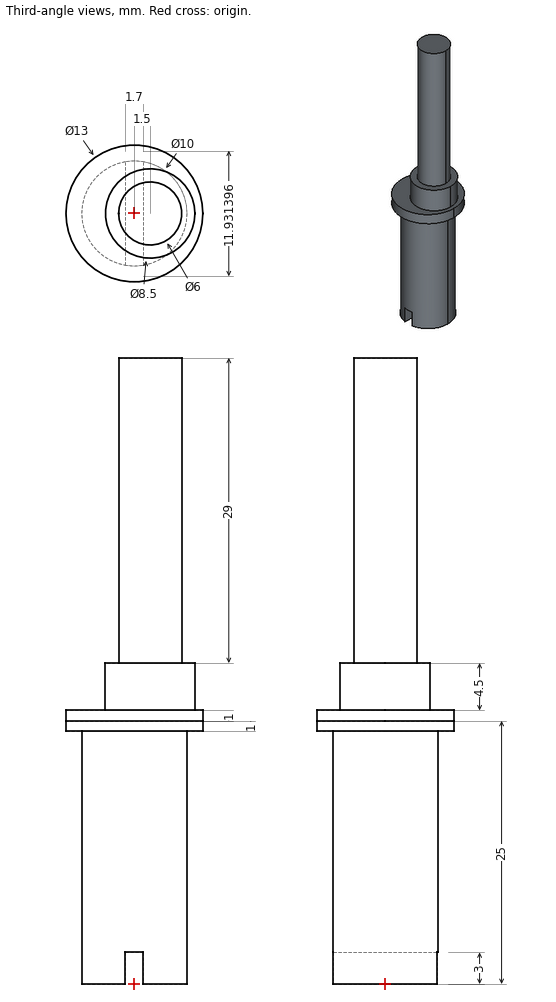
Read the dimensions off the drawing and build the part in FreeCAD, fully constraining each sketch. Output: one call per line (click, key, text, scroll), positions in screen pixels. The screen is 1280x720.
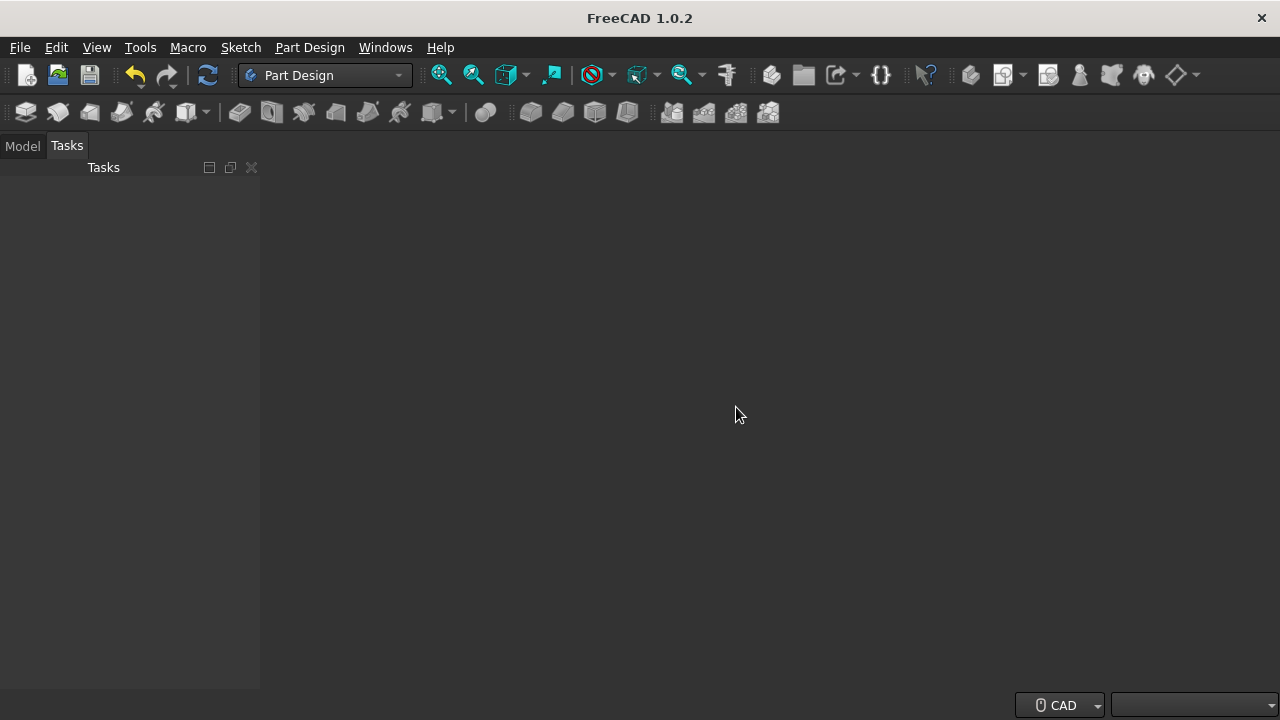
click(26, 76)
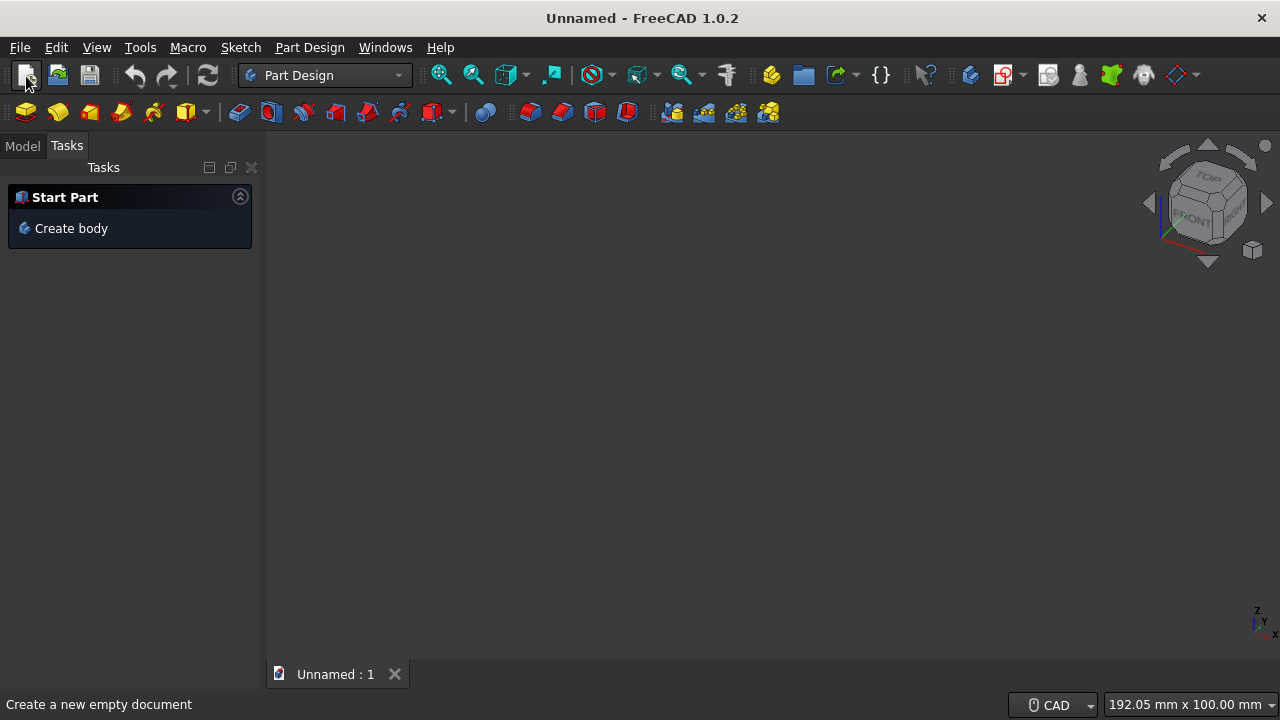
click(1004, 76)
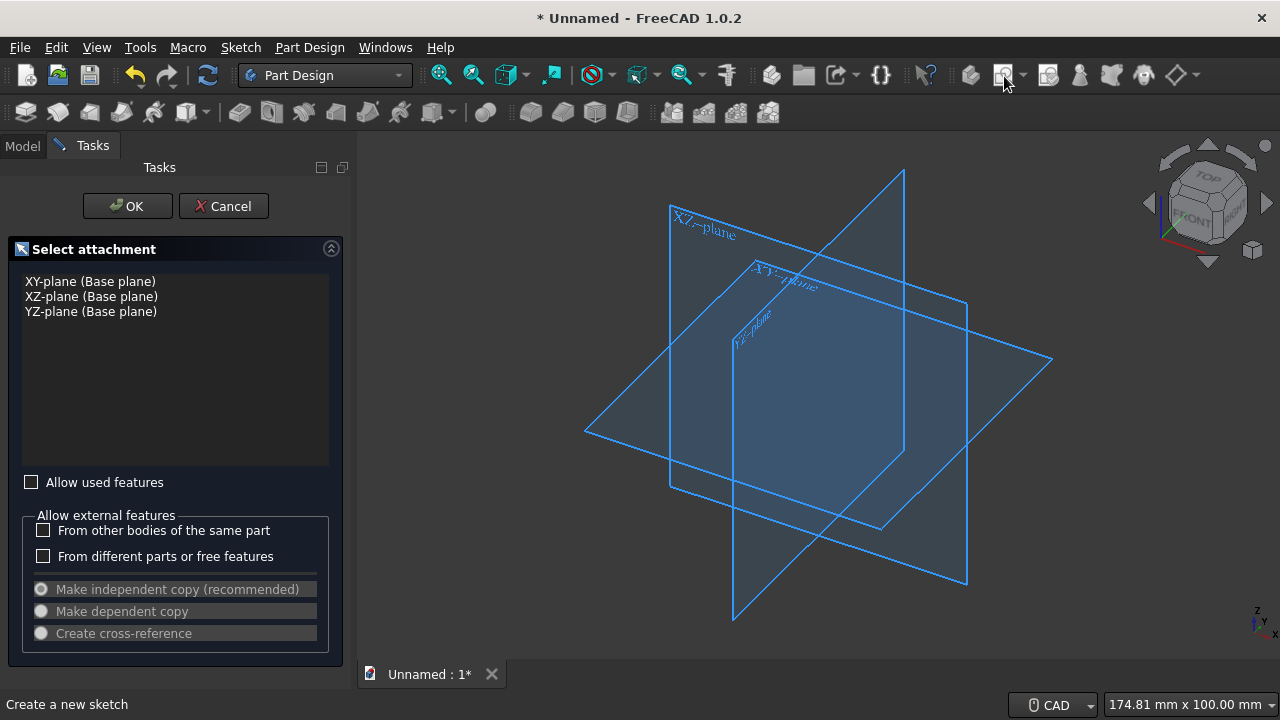
click(82, 282)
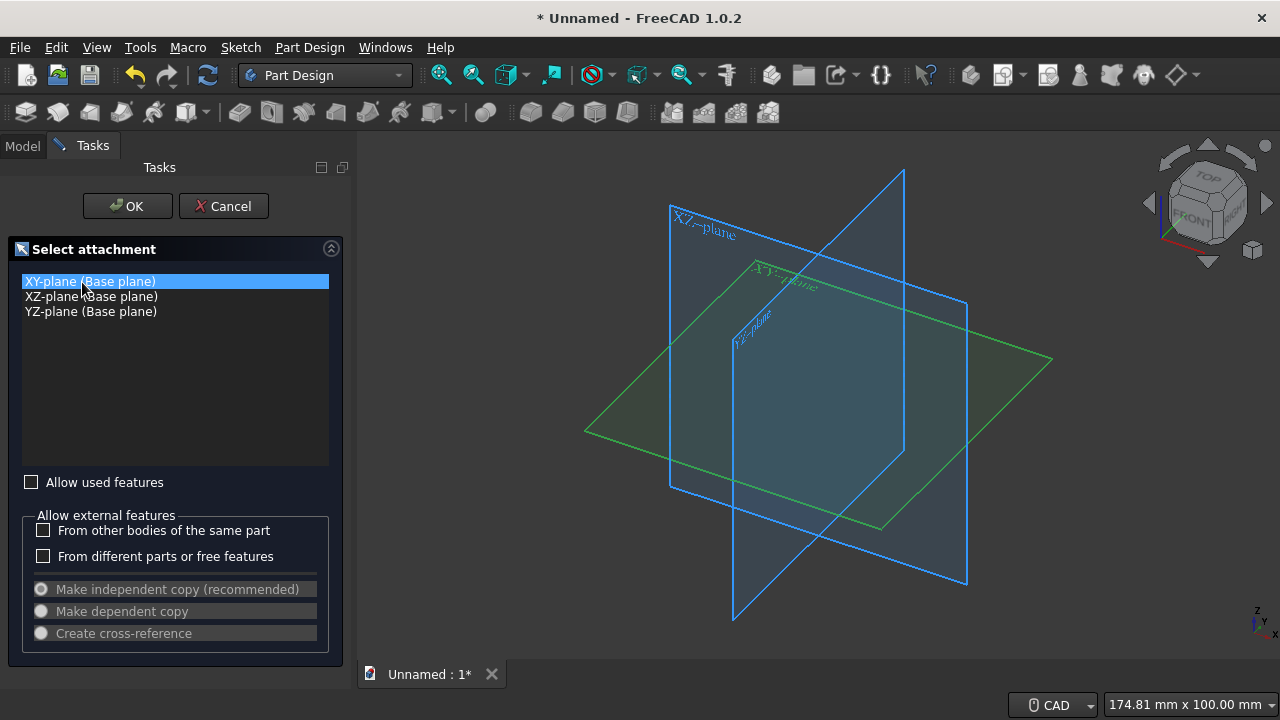
click(128, 206)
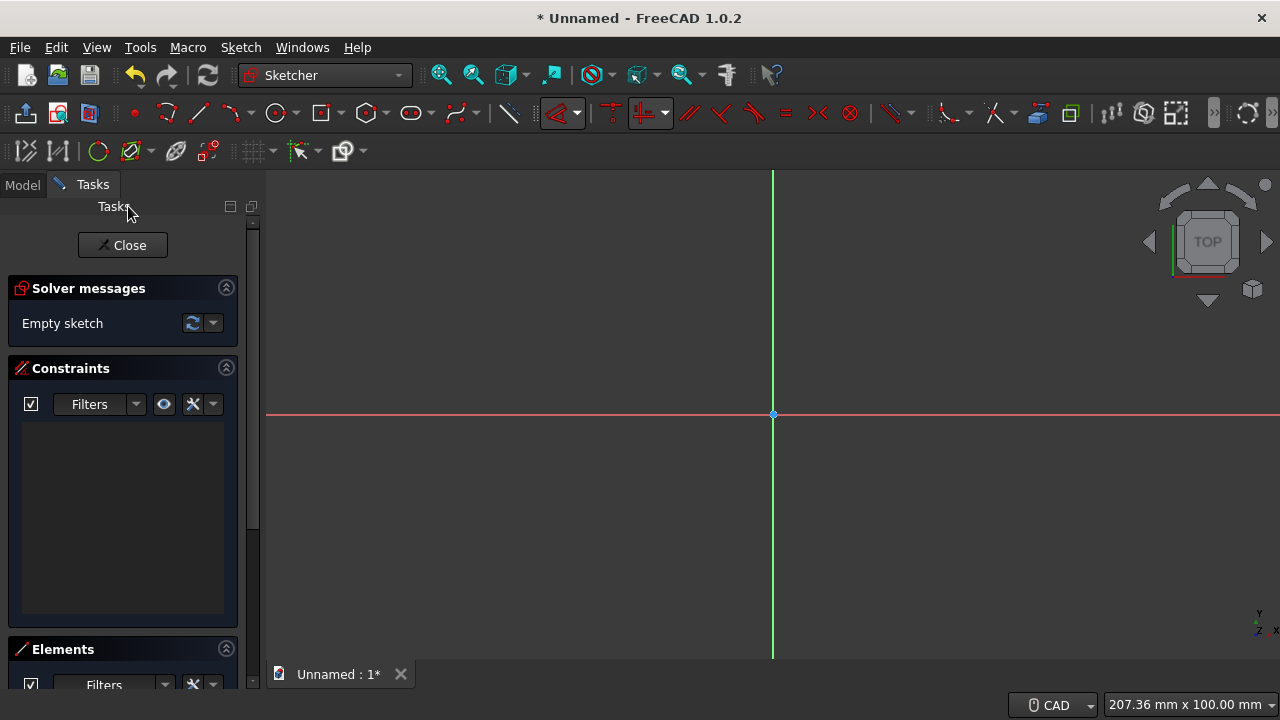
scroll(787, 414, up, 9)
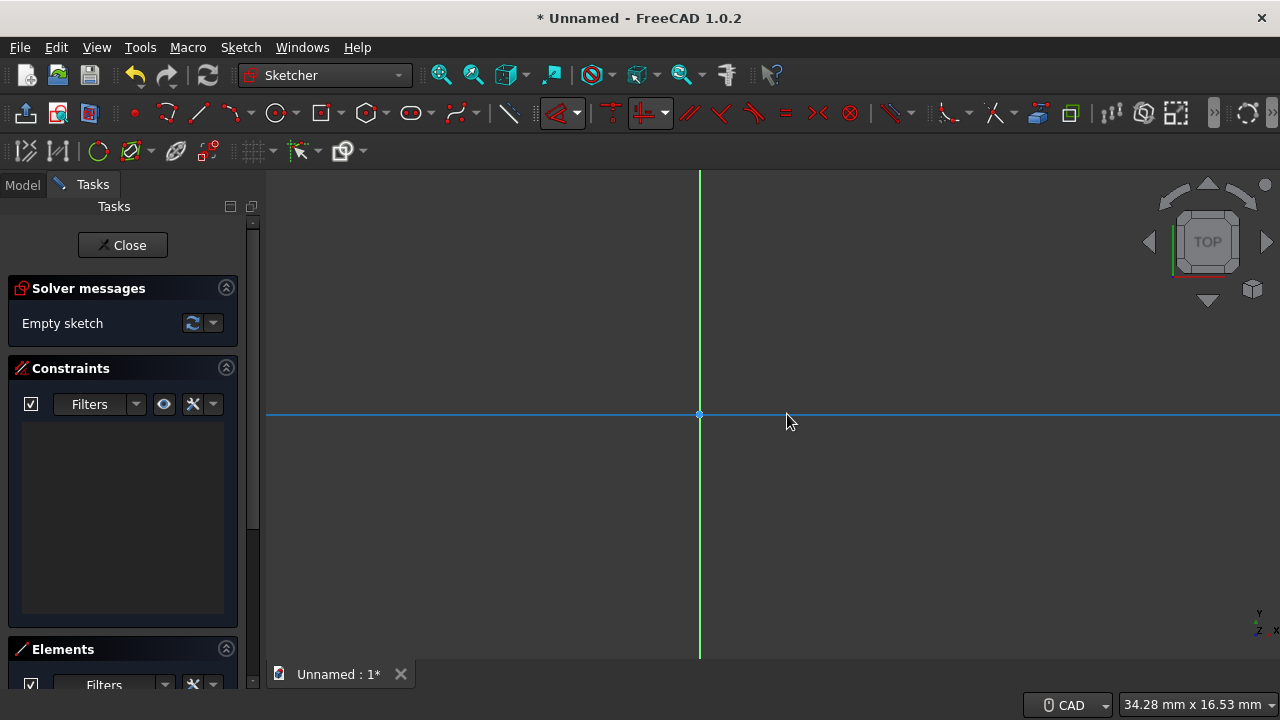
click(276, 114)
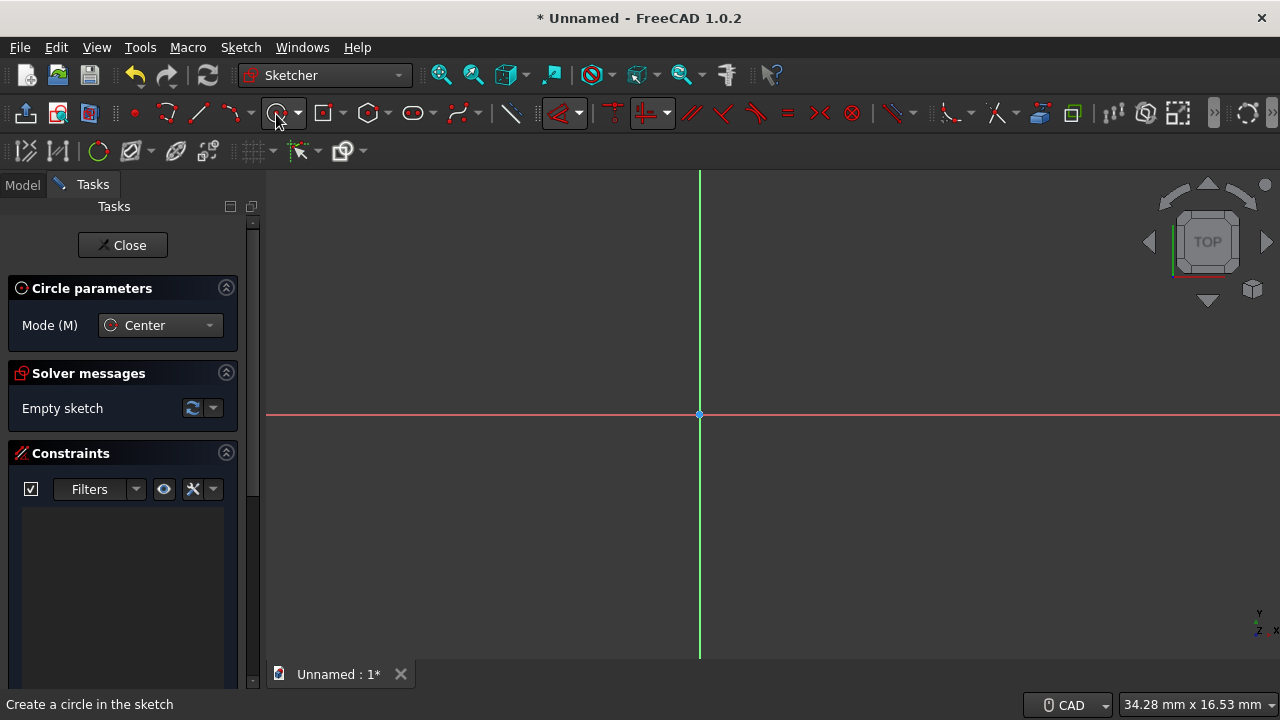
click(700, 414)
move(804, 310)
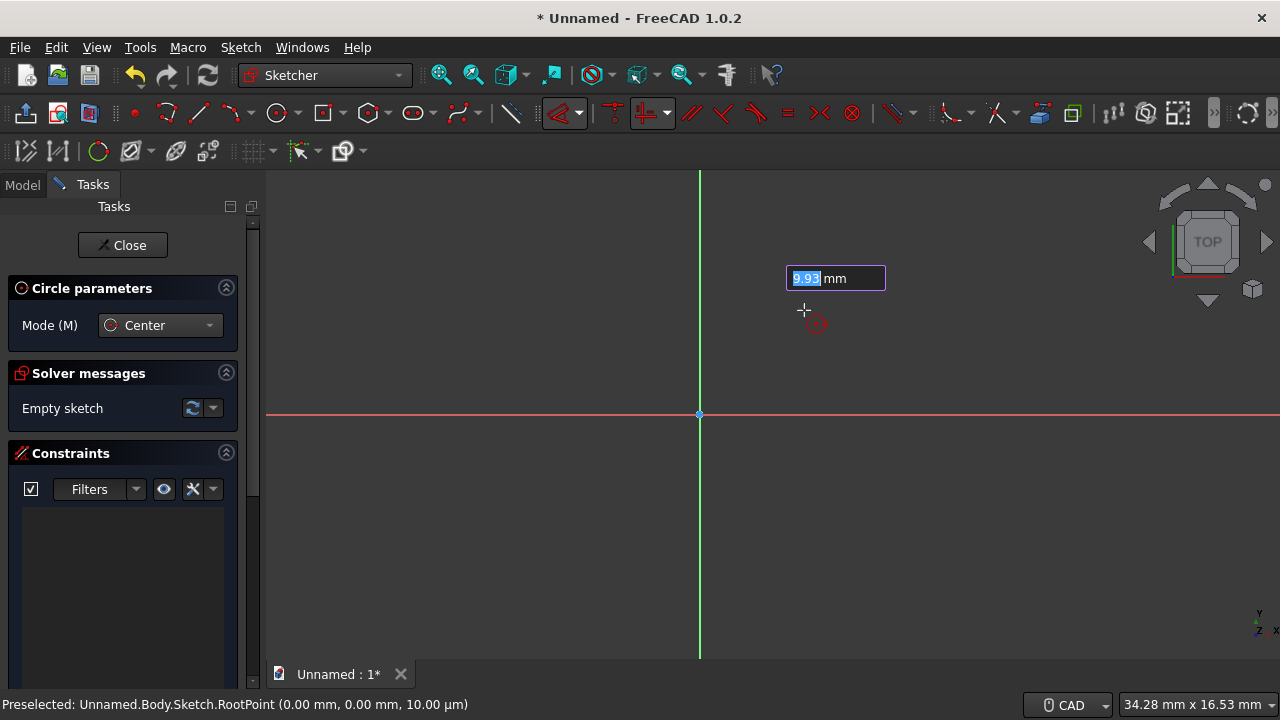
text(10)
key(Return)
key(Escape)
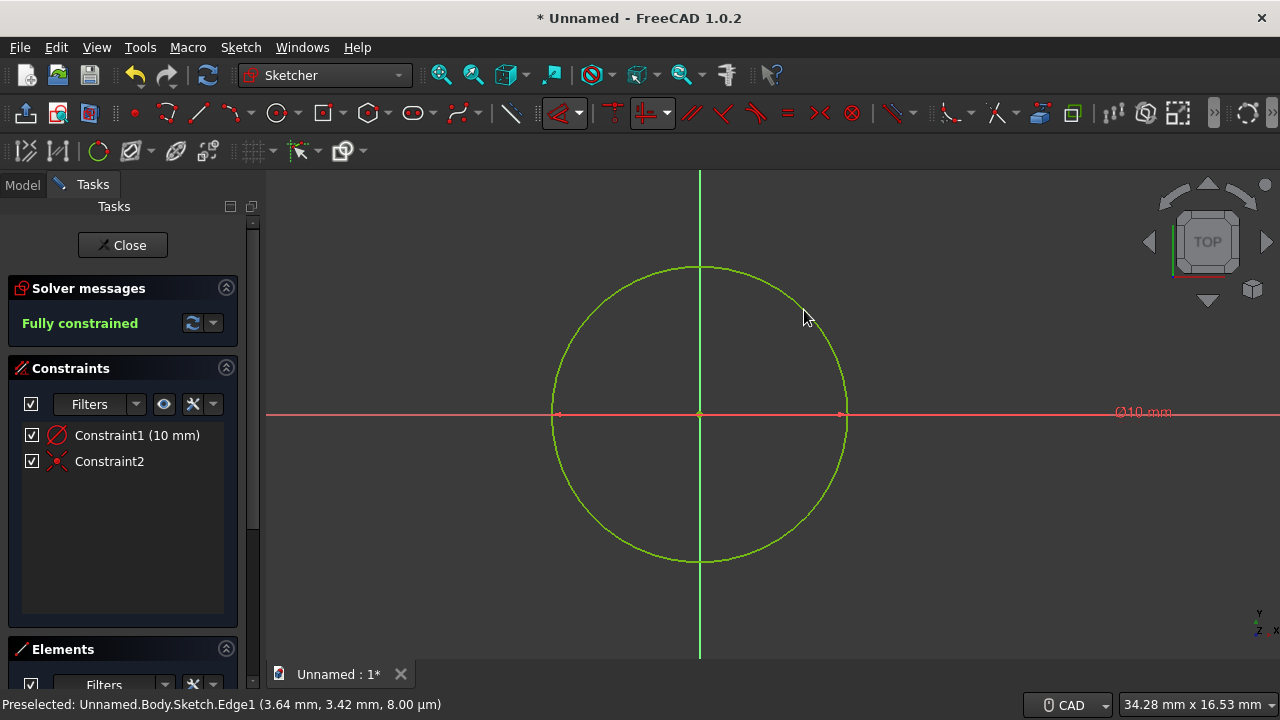
click(123, 245)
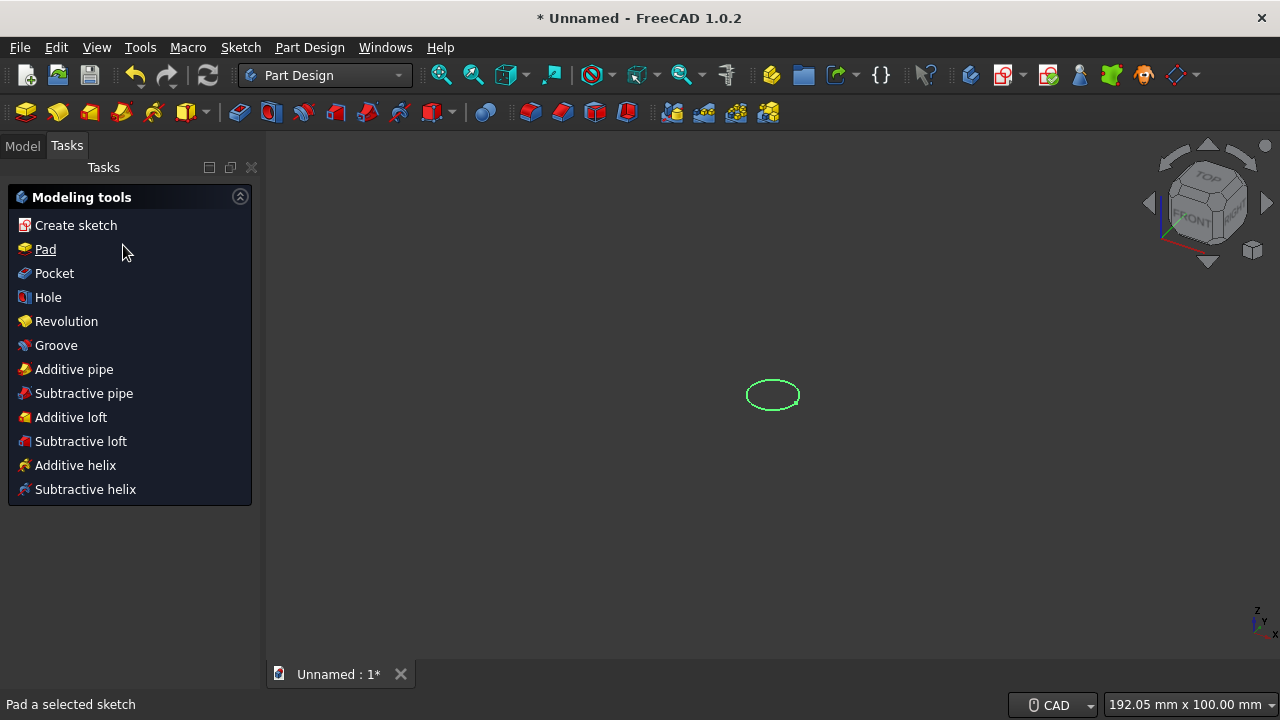
click(26, 112)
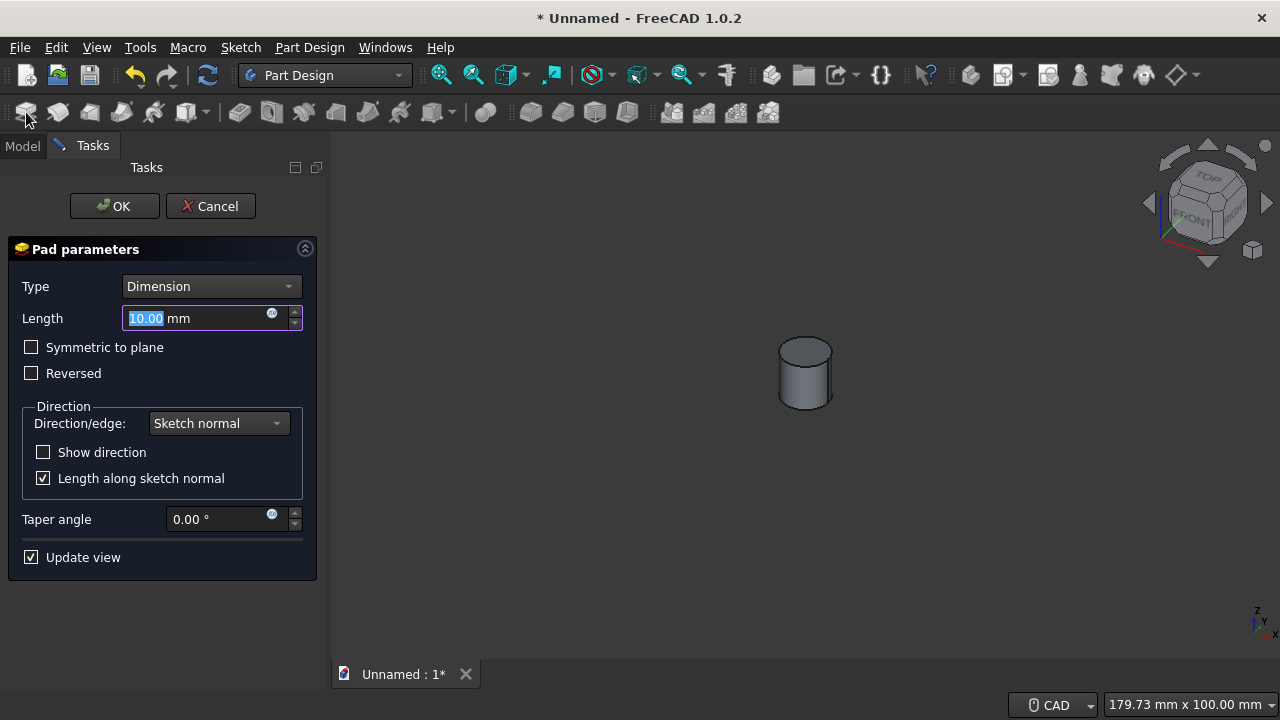
text(25)
key(Tab)